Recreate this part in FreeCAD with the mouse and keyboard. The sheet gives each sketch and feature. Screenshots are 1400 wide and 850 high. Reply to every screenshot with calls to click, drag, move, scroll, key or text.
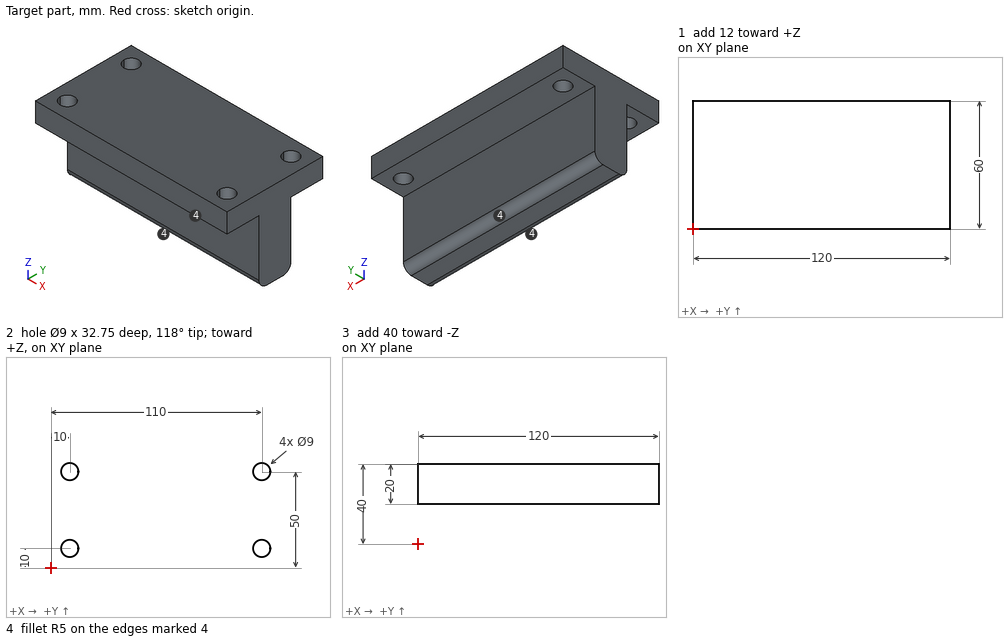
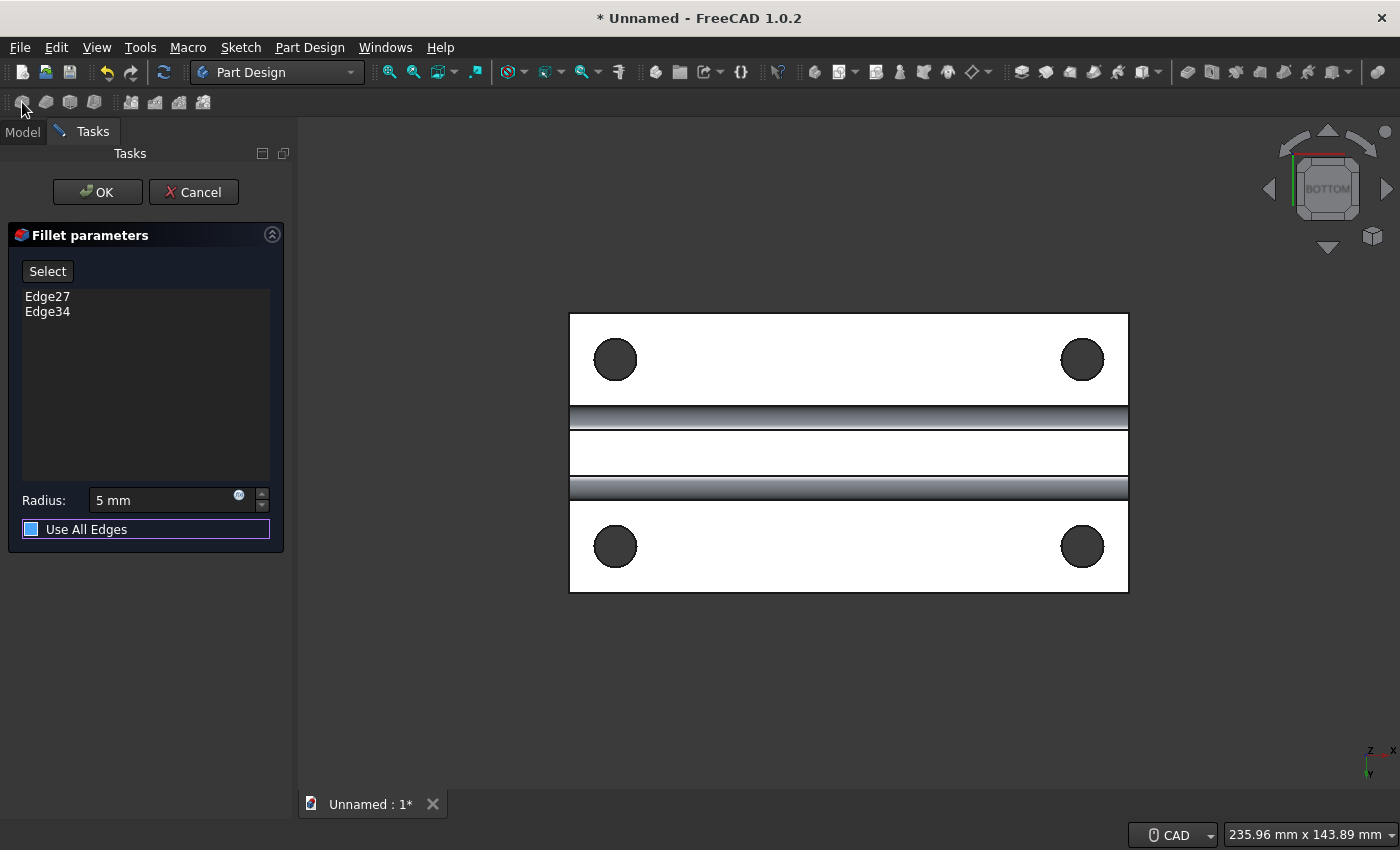
click(98, 192)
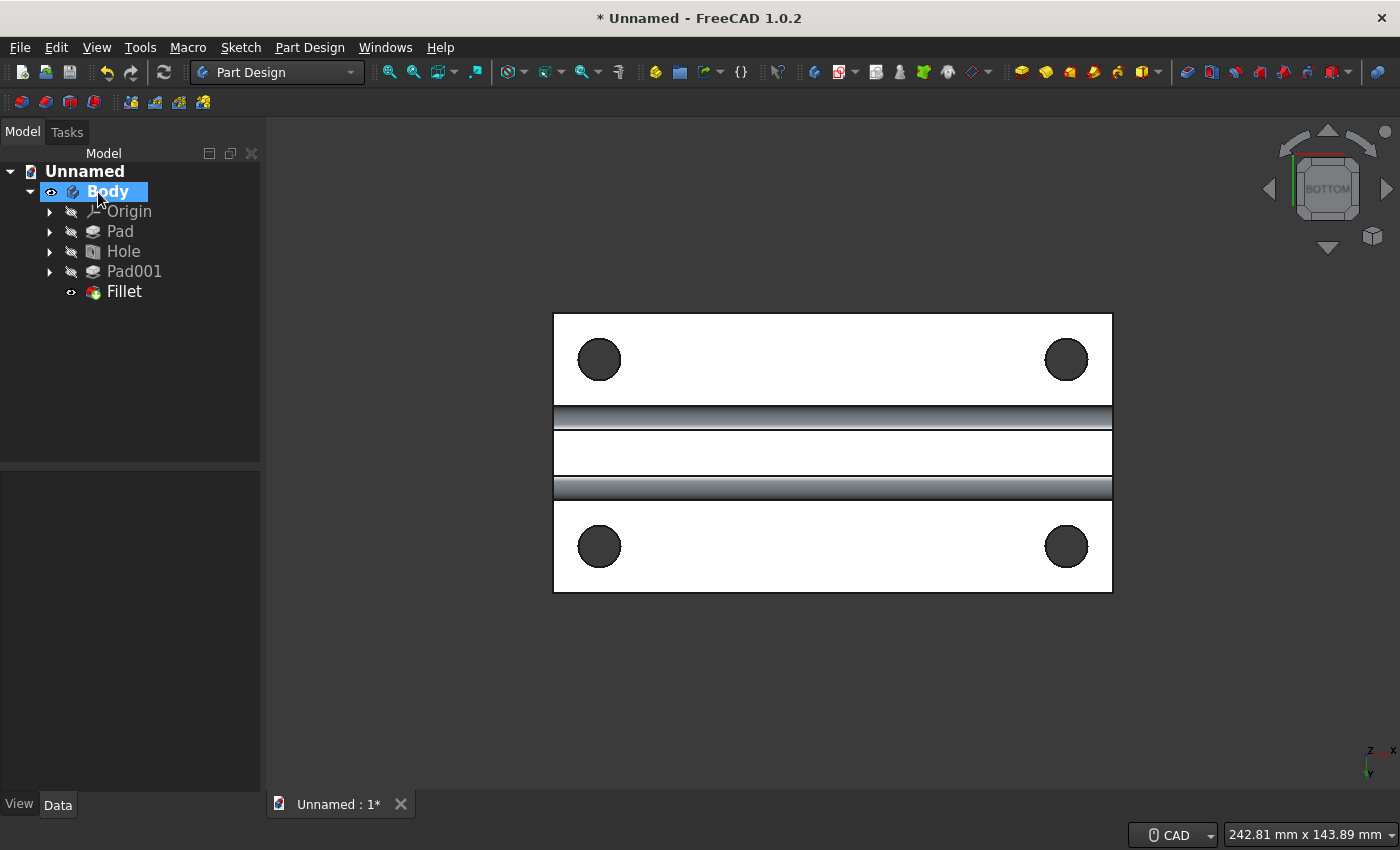
key(0)